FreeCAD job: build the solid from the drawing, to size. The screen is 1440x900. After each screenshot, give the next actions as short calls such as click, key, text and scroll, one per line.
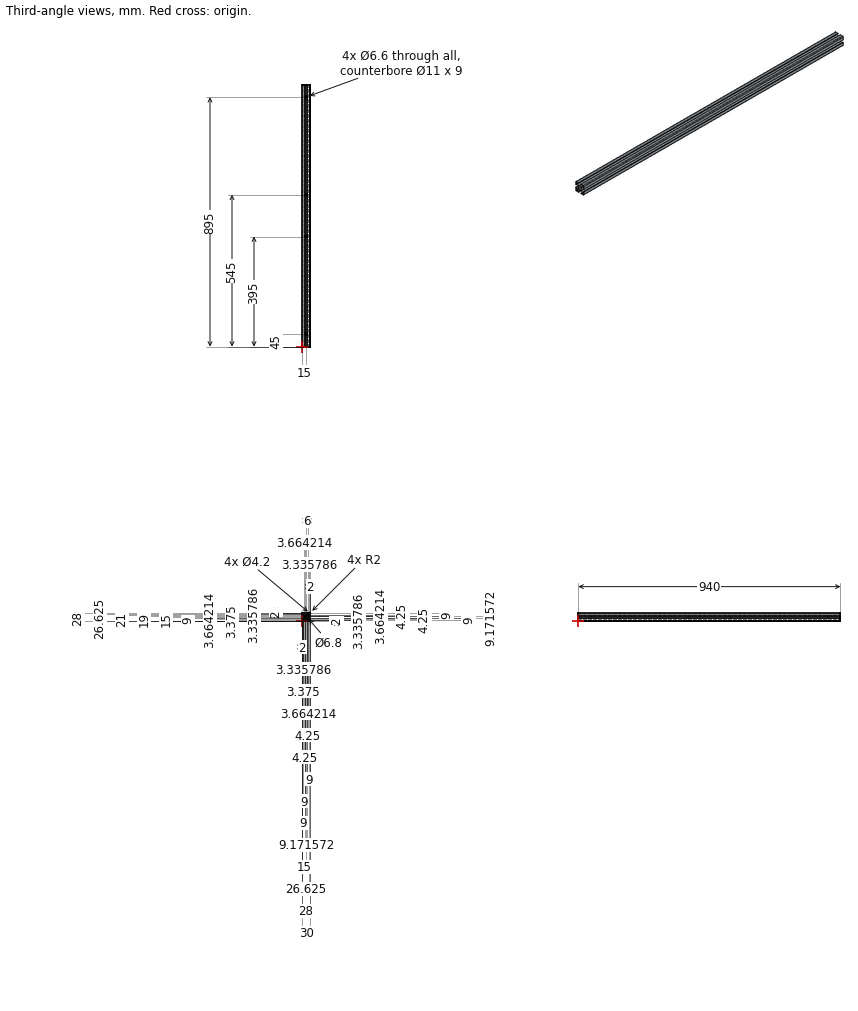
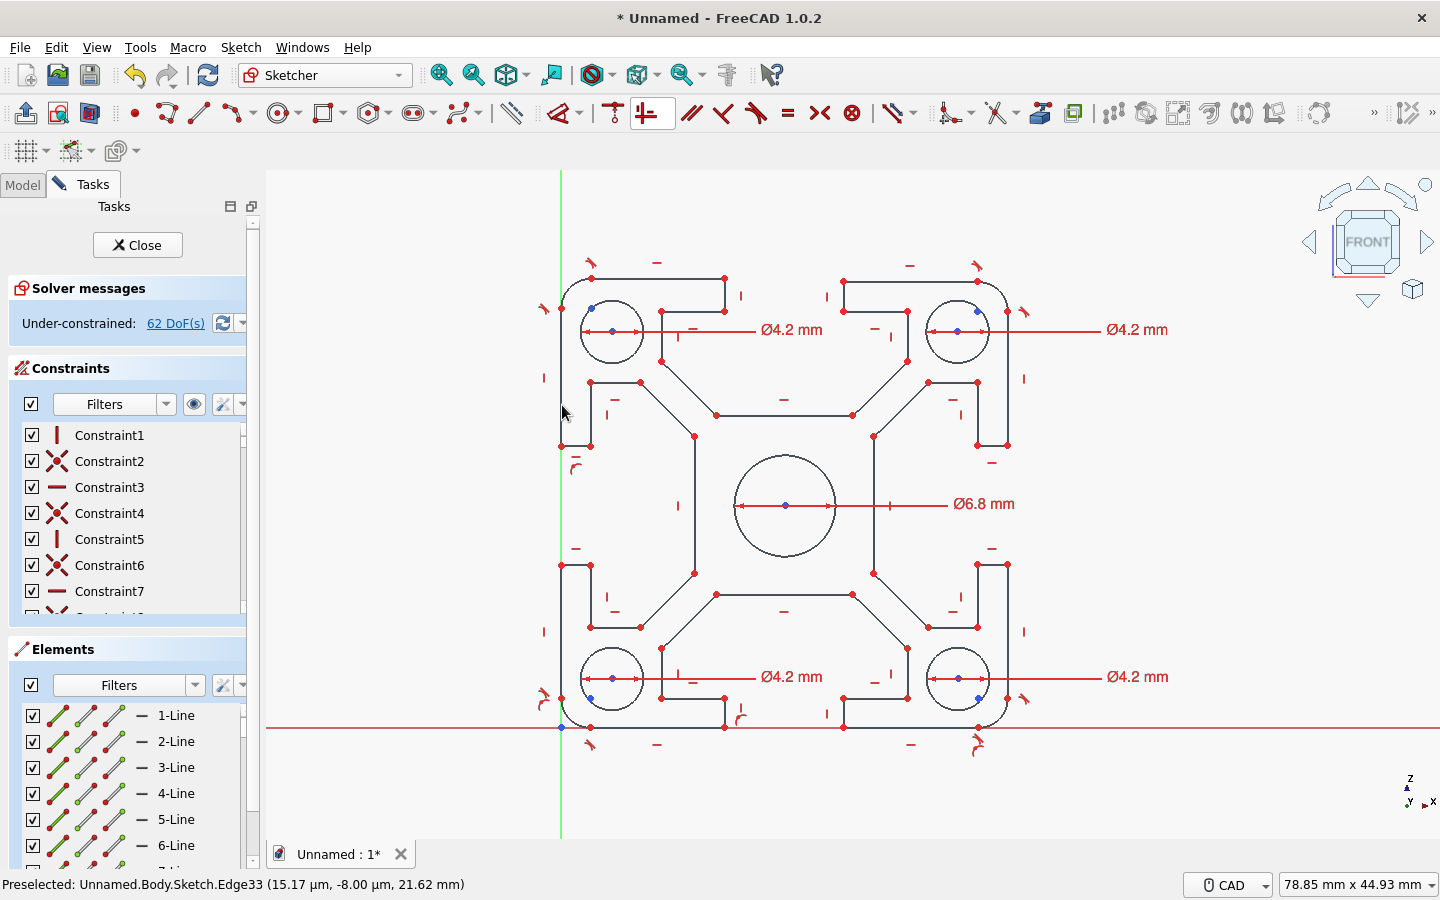
click(992, 725)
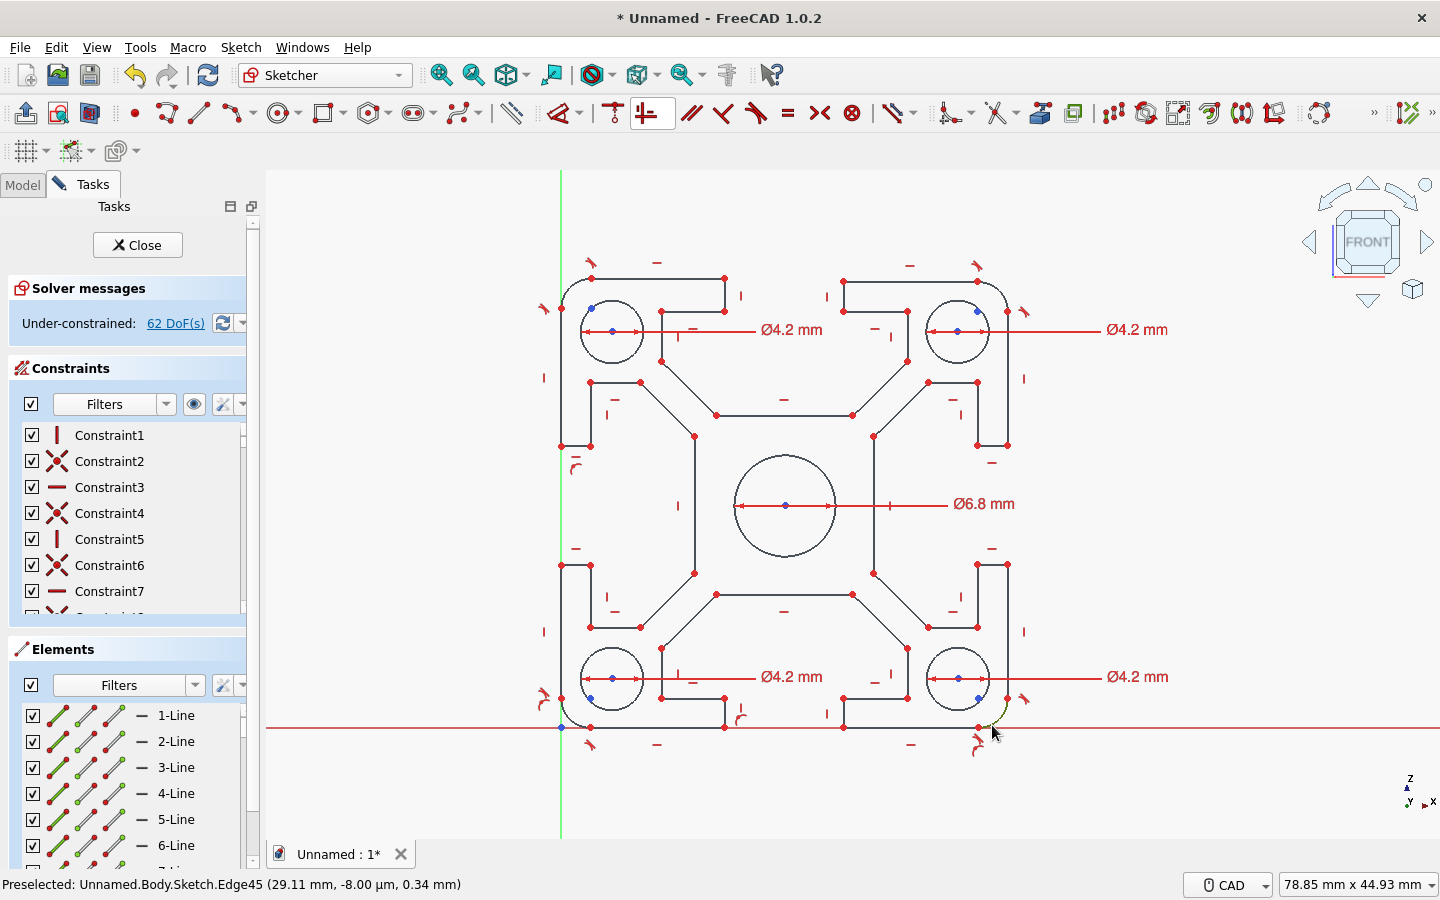
click(565, 712)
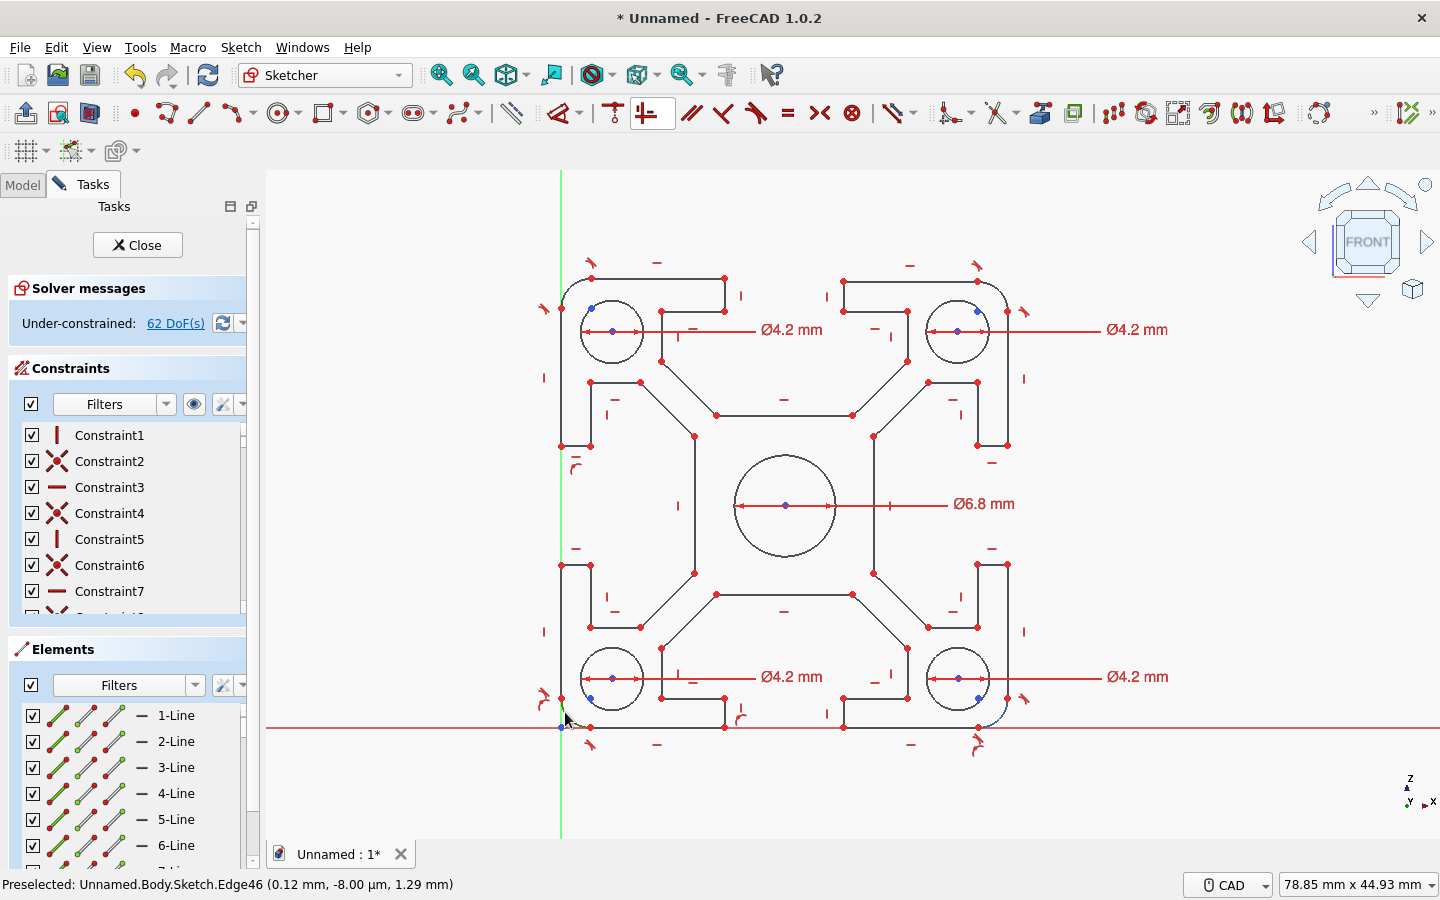
click(578, 282)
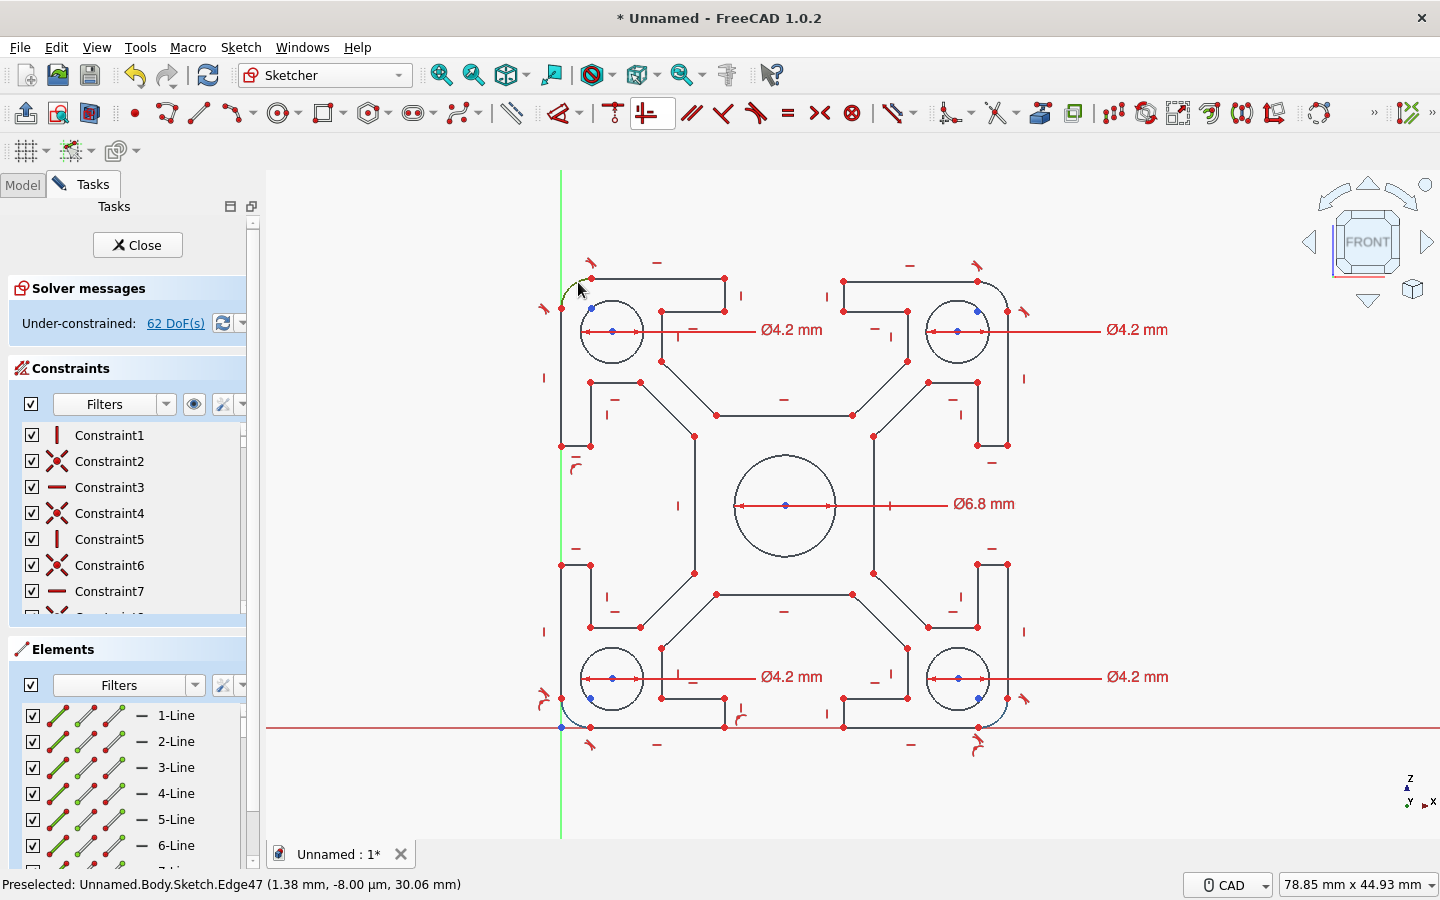
click(1005, 298)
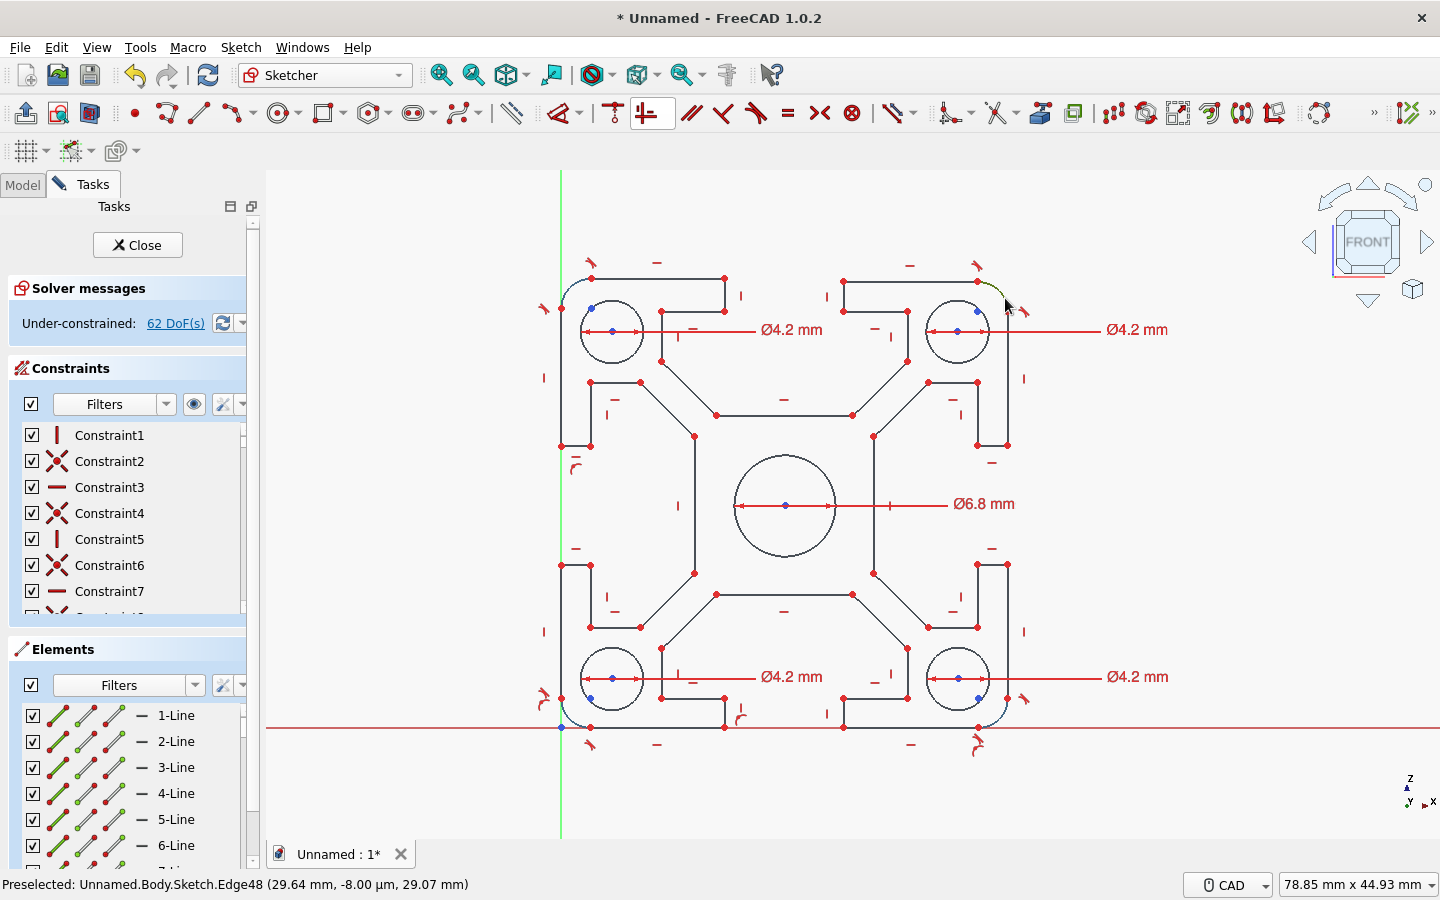
click(788, 114)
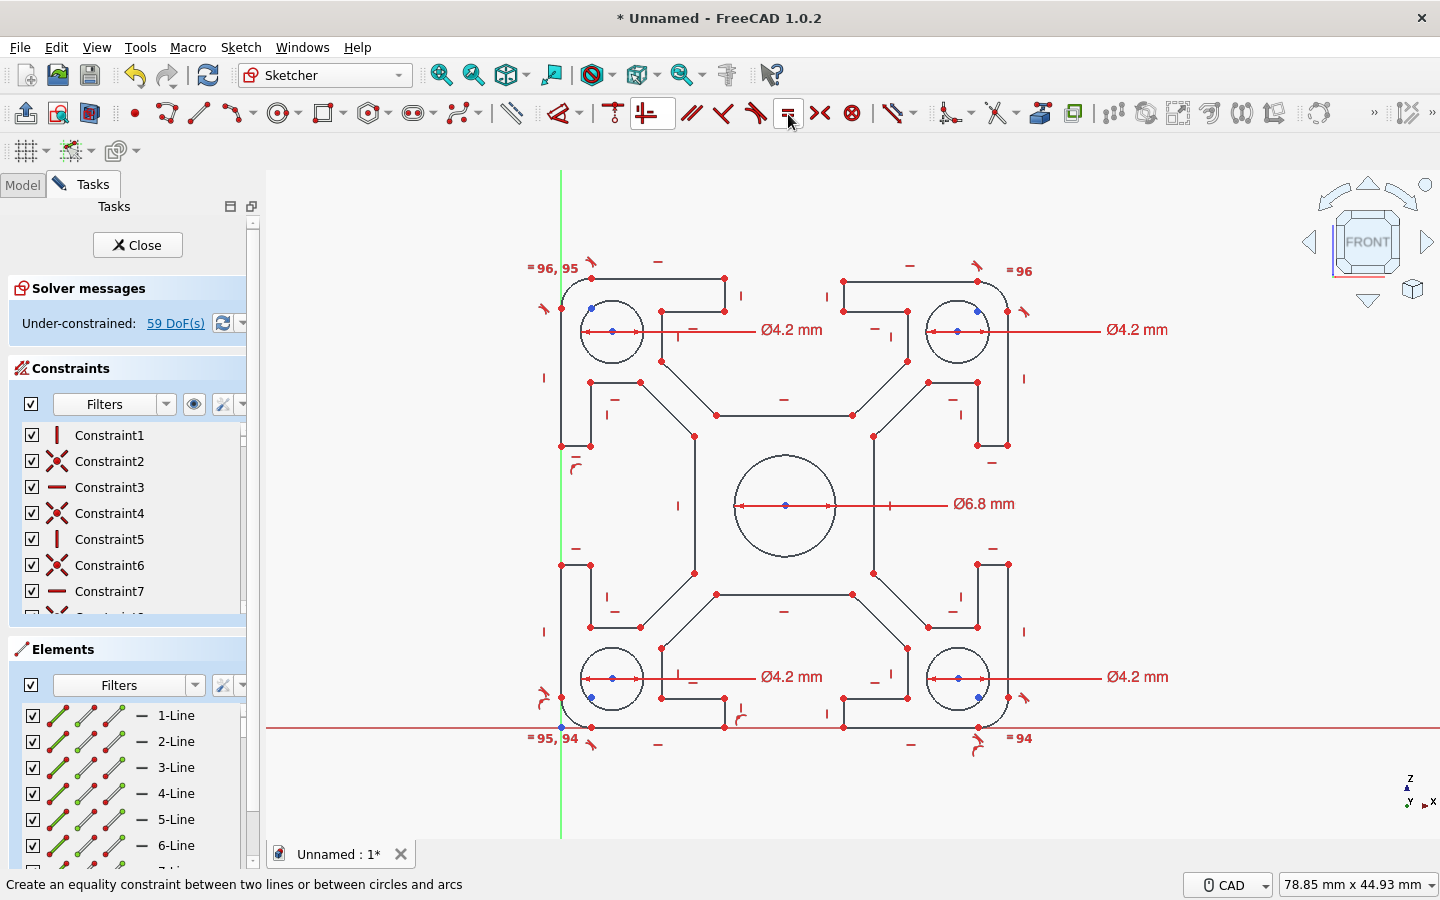
click(558, 114)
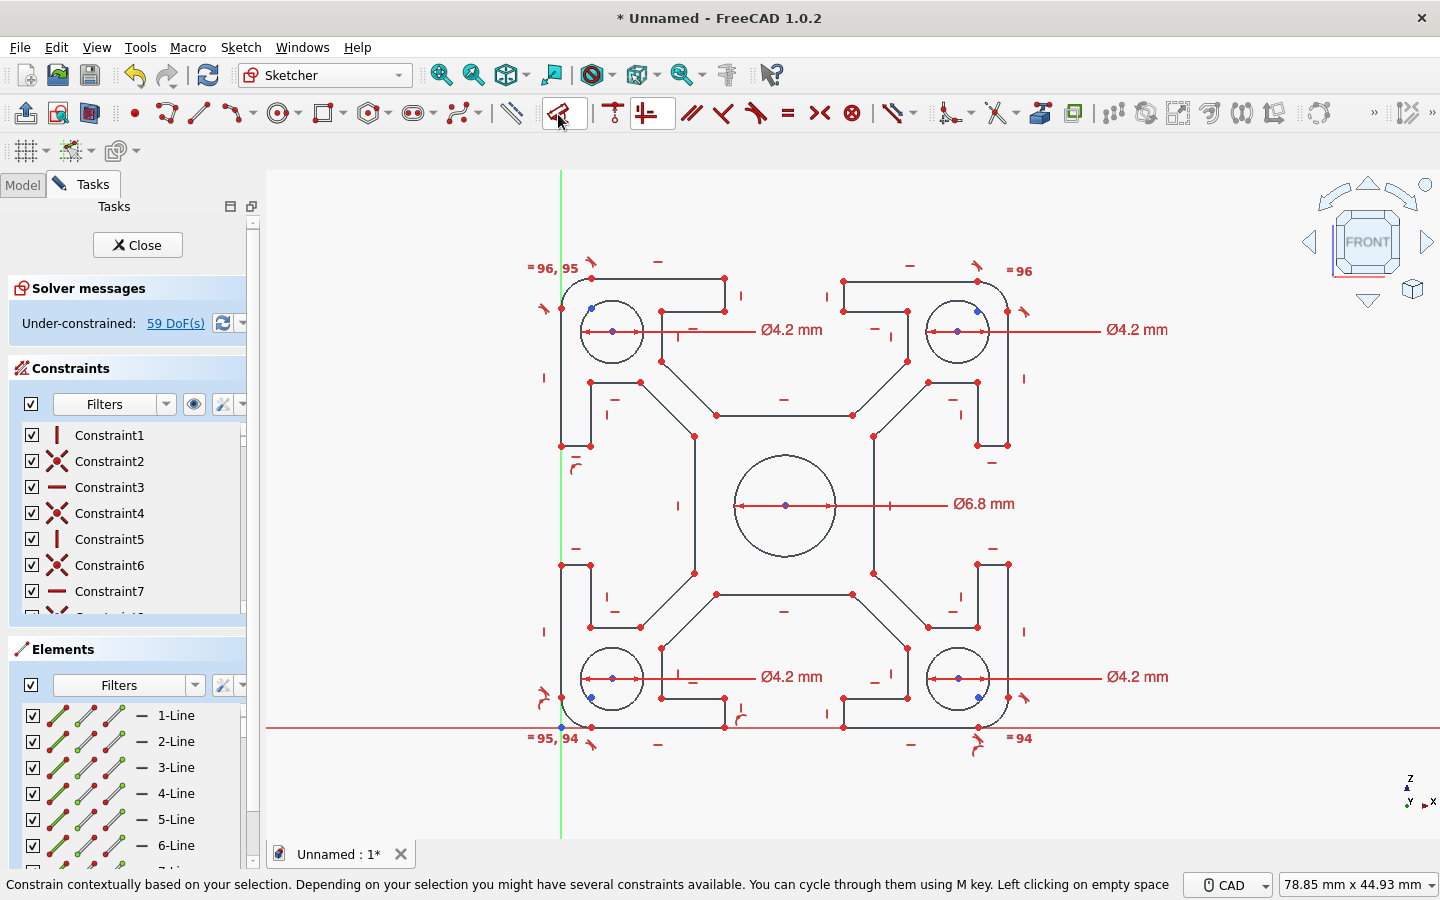
scroll(992, 725, up, 2)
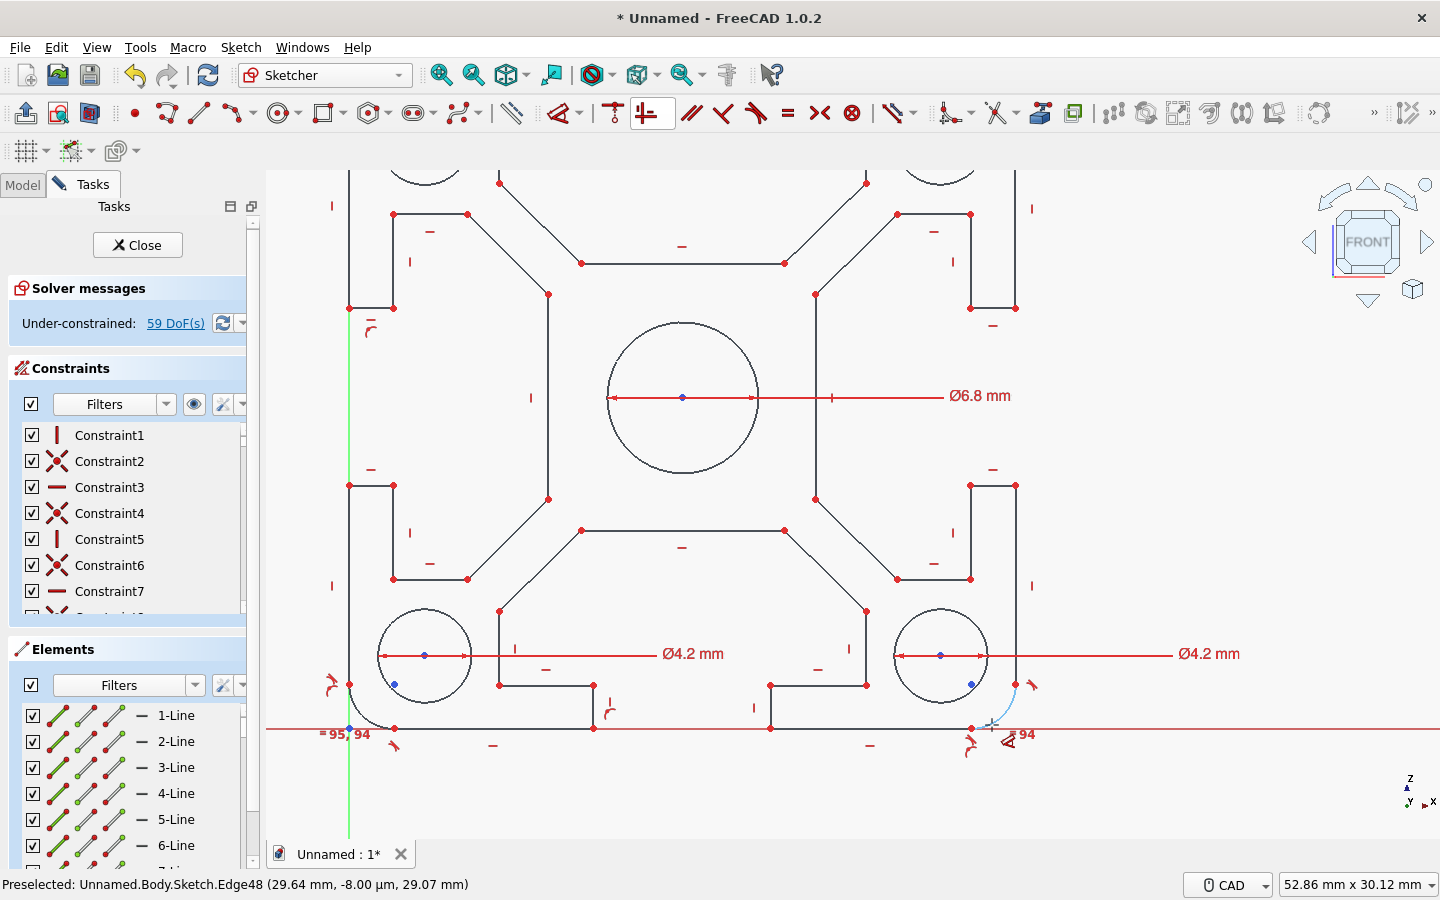
click(991, 724)
click(1005, 753)